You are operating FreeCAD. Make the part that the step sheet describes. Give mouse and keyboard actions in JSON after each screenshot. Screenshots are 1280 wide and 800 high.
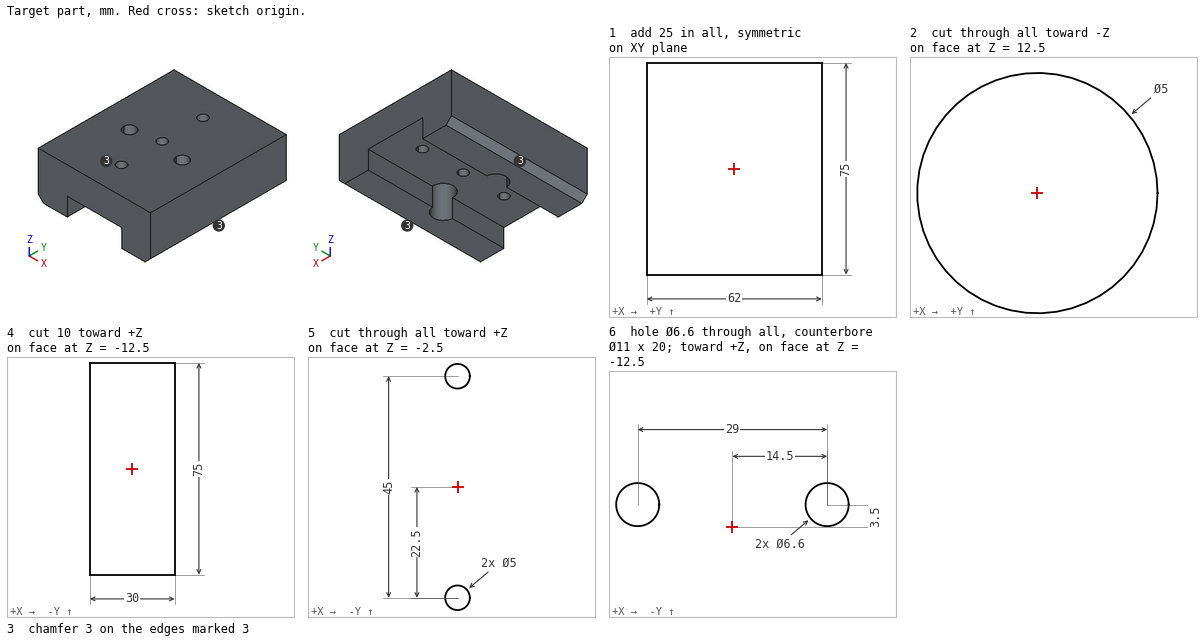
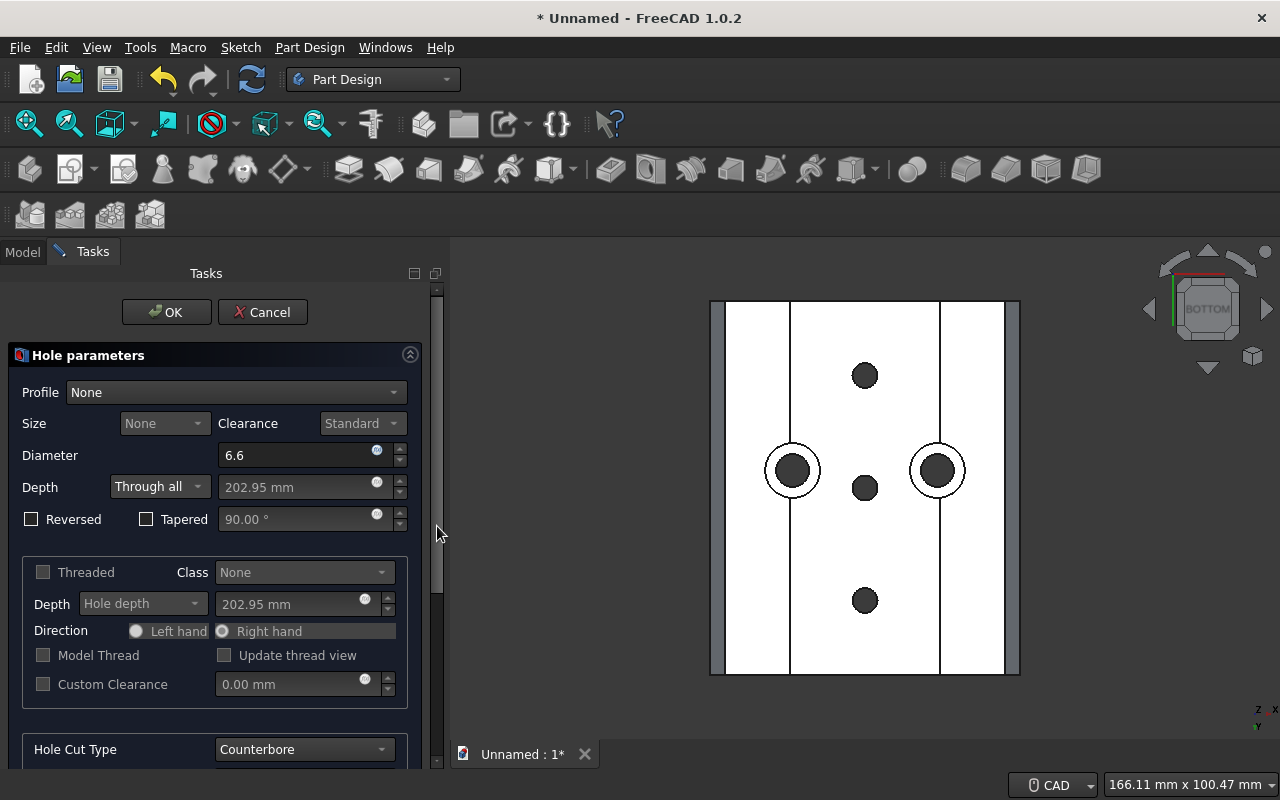
{"action": "left_click", "coordinate": [167, 312]}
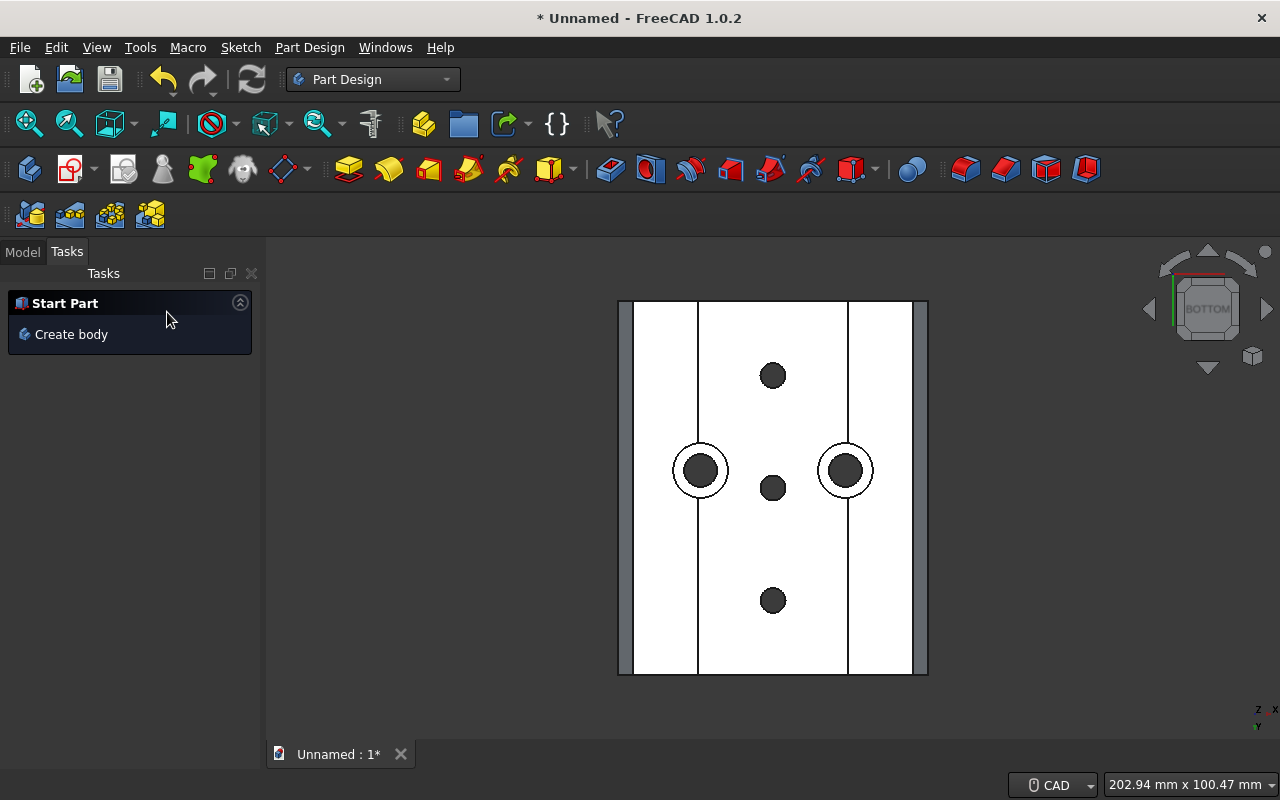
{"action": "key", "text": "0"}